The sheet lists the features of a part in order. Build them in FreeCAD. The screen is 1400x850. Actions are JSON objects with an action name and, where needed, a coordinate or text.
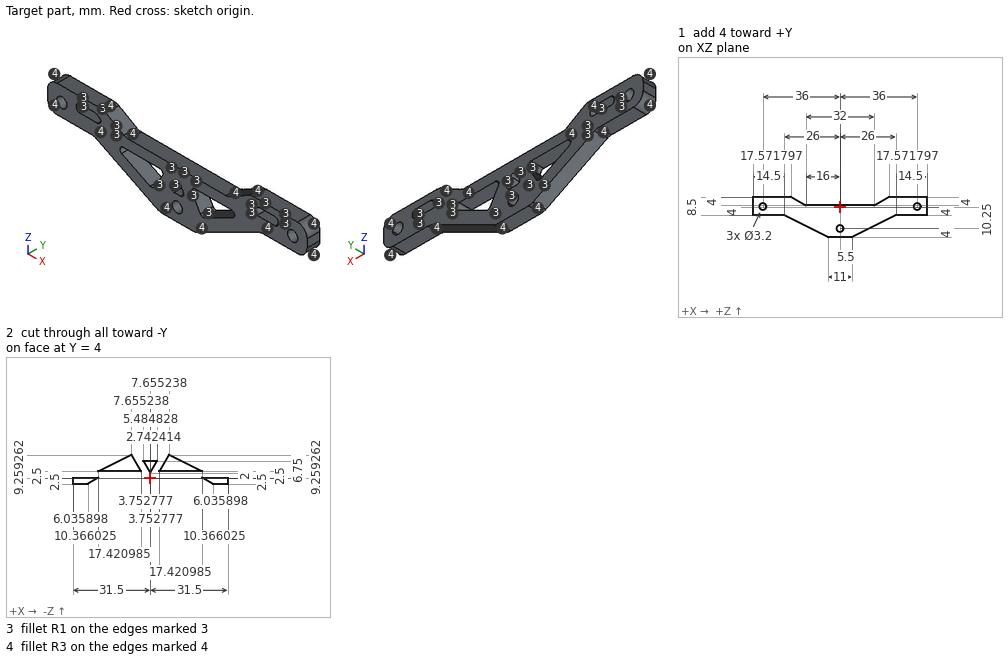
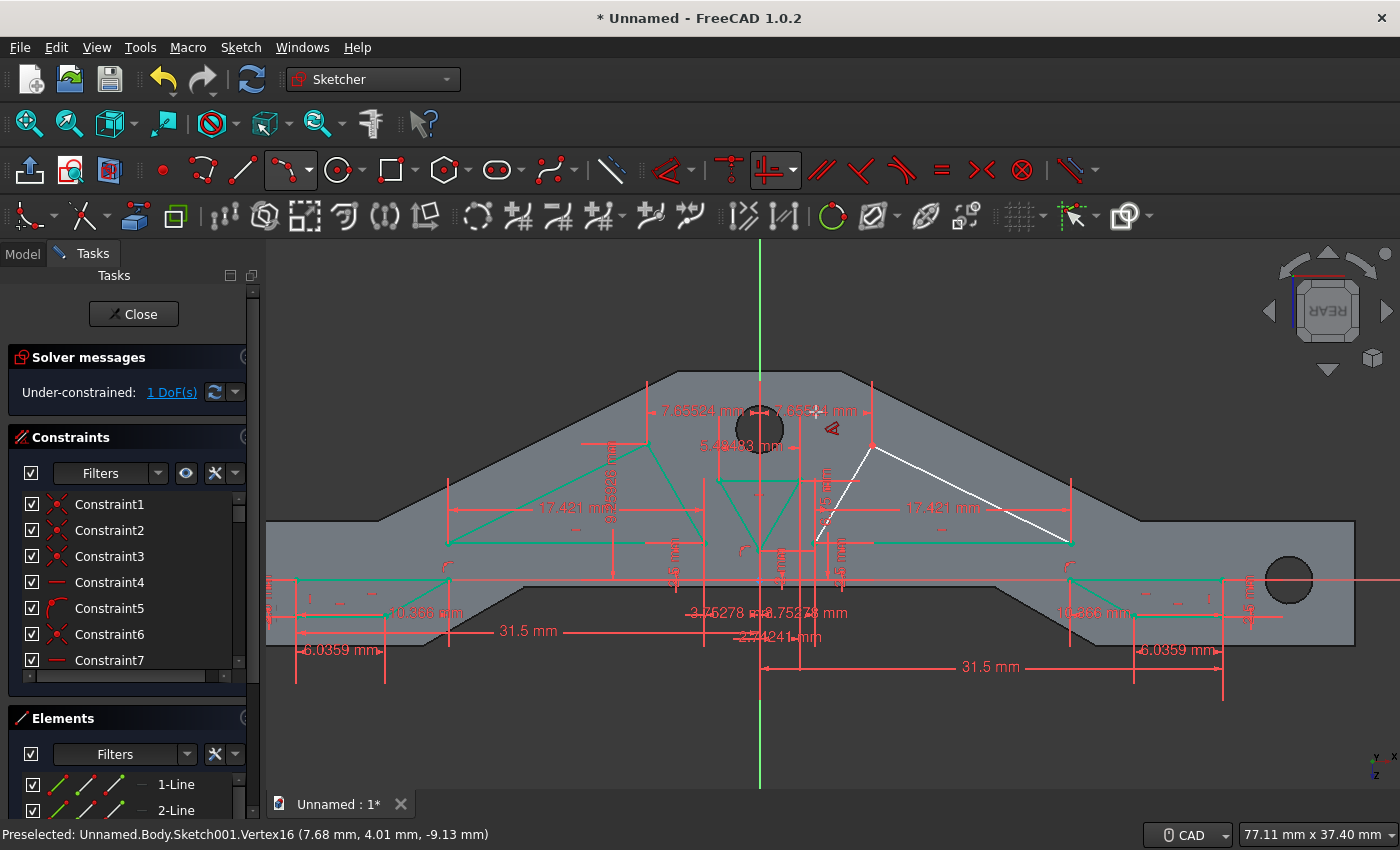
{"action": "left_click", "coordinate": [872, 446]}
{"action": "left_click", "coordinate": [906, 482]}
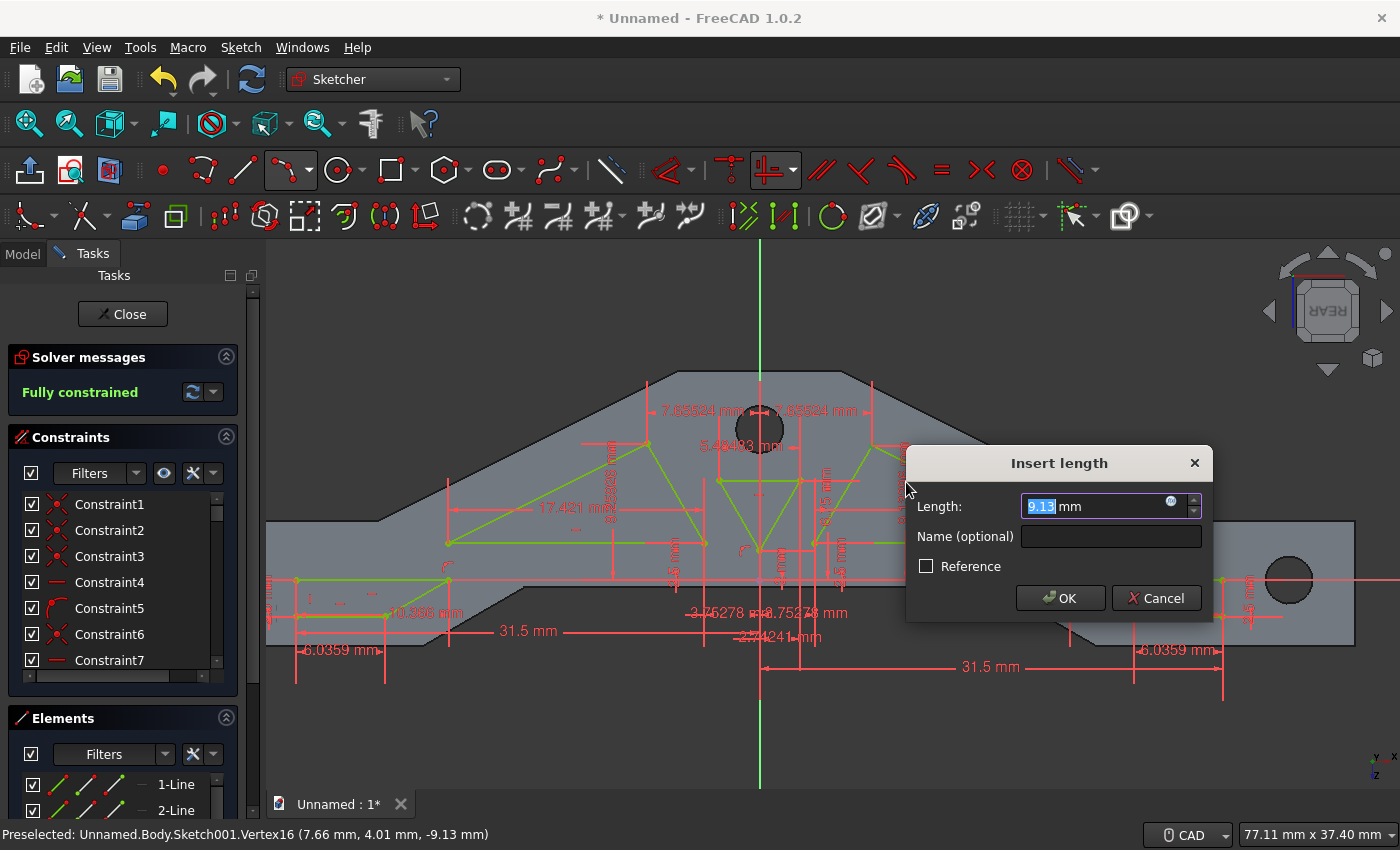
{"action": "type", "text": "9.259262"}
{"action": "key", "text": "Return"}
{"action": "key", "text": "Escape"}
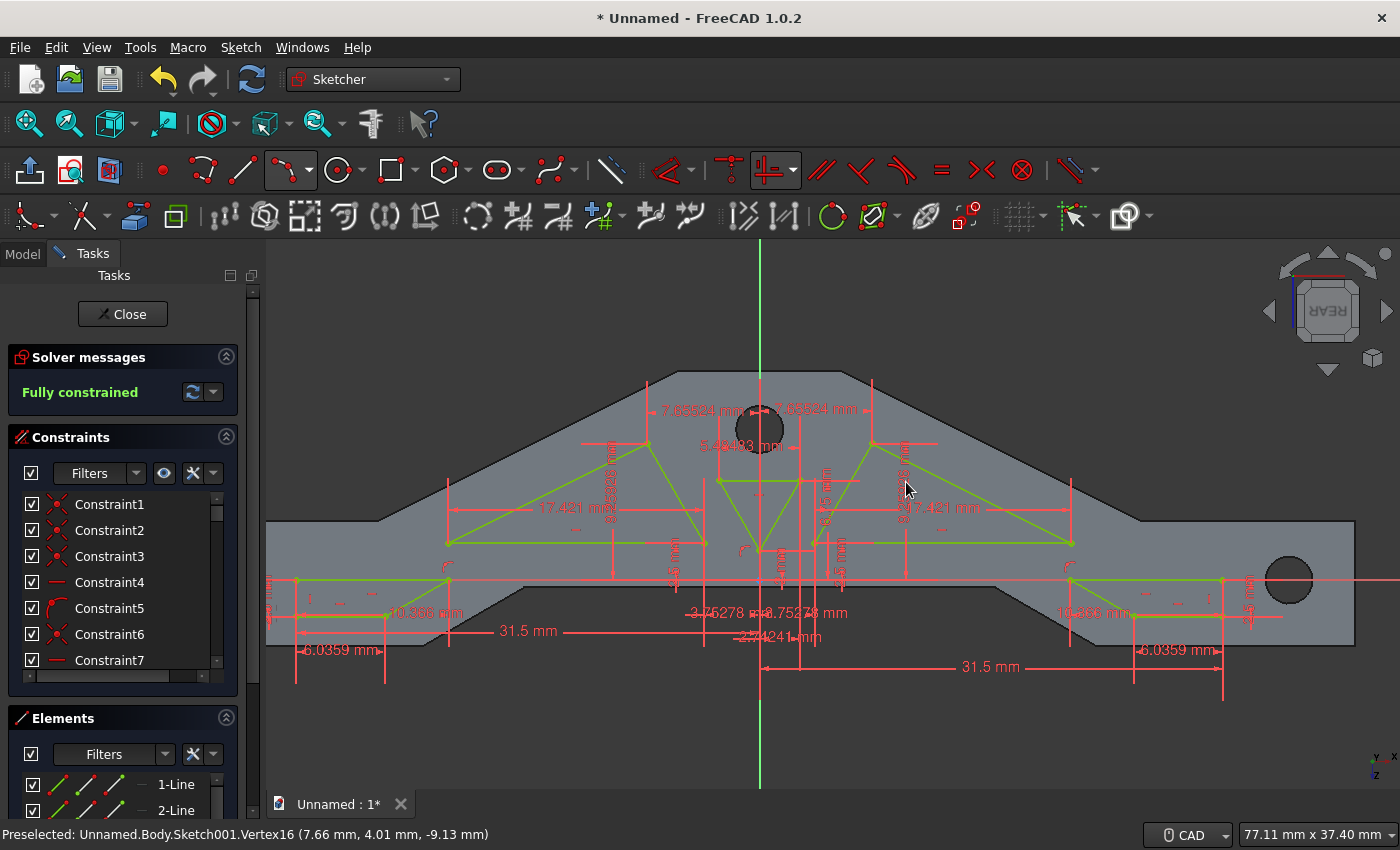
{"action": "left_click", "coordinate": [123, 314]}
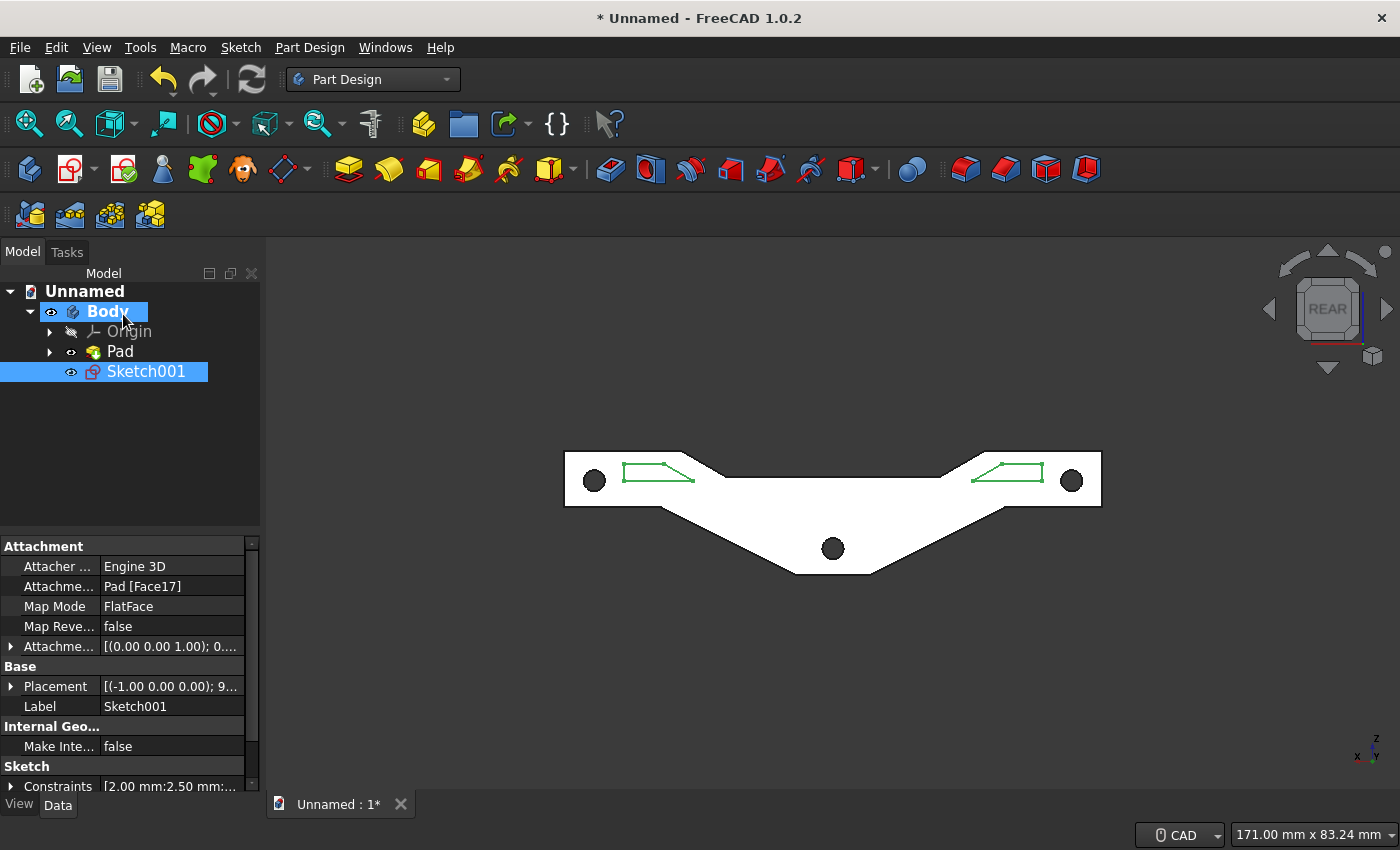
{"action": "left_click", "coordinate": [612, 170]}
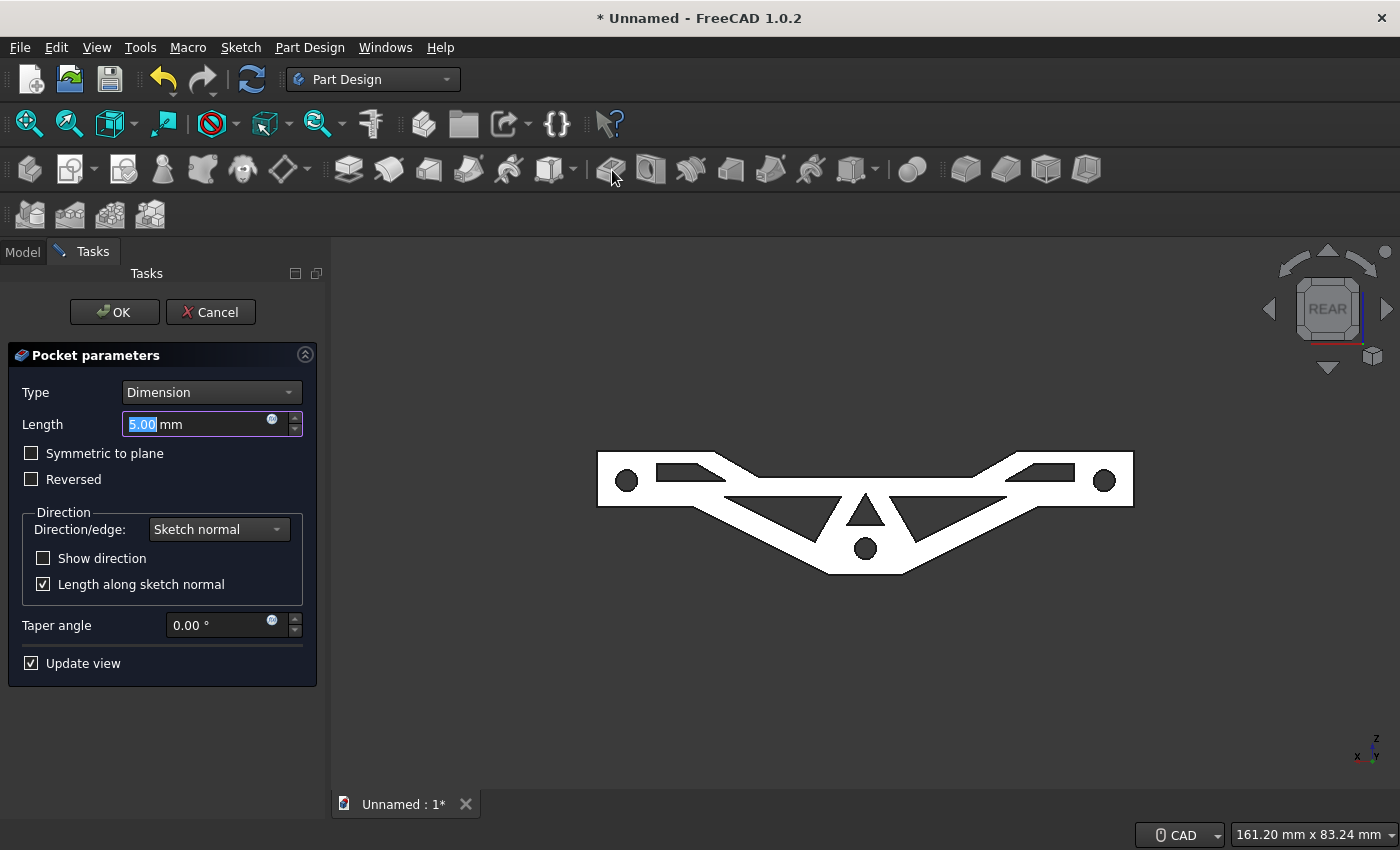
{"action": "left_click", "coordinate": [212, 392]}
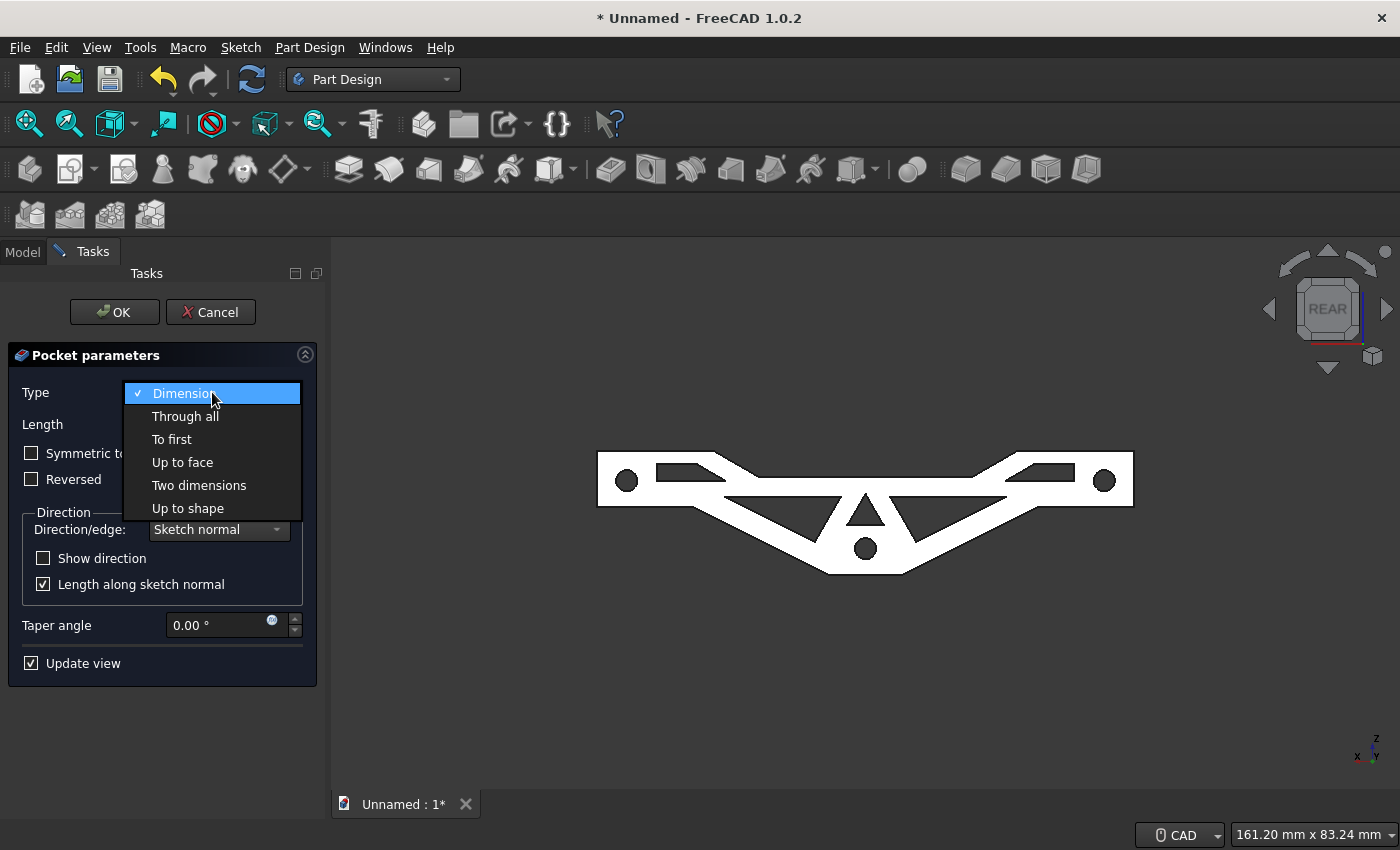
{"action": "left_click", "coordinate": [212, 416]}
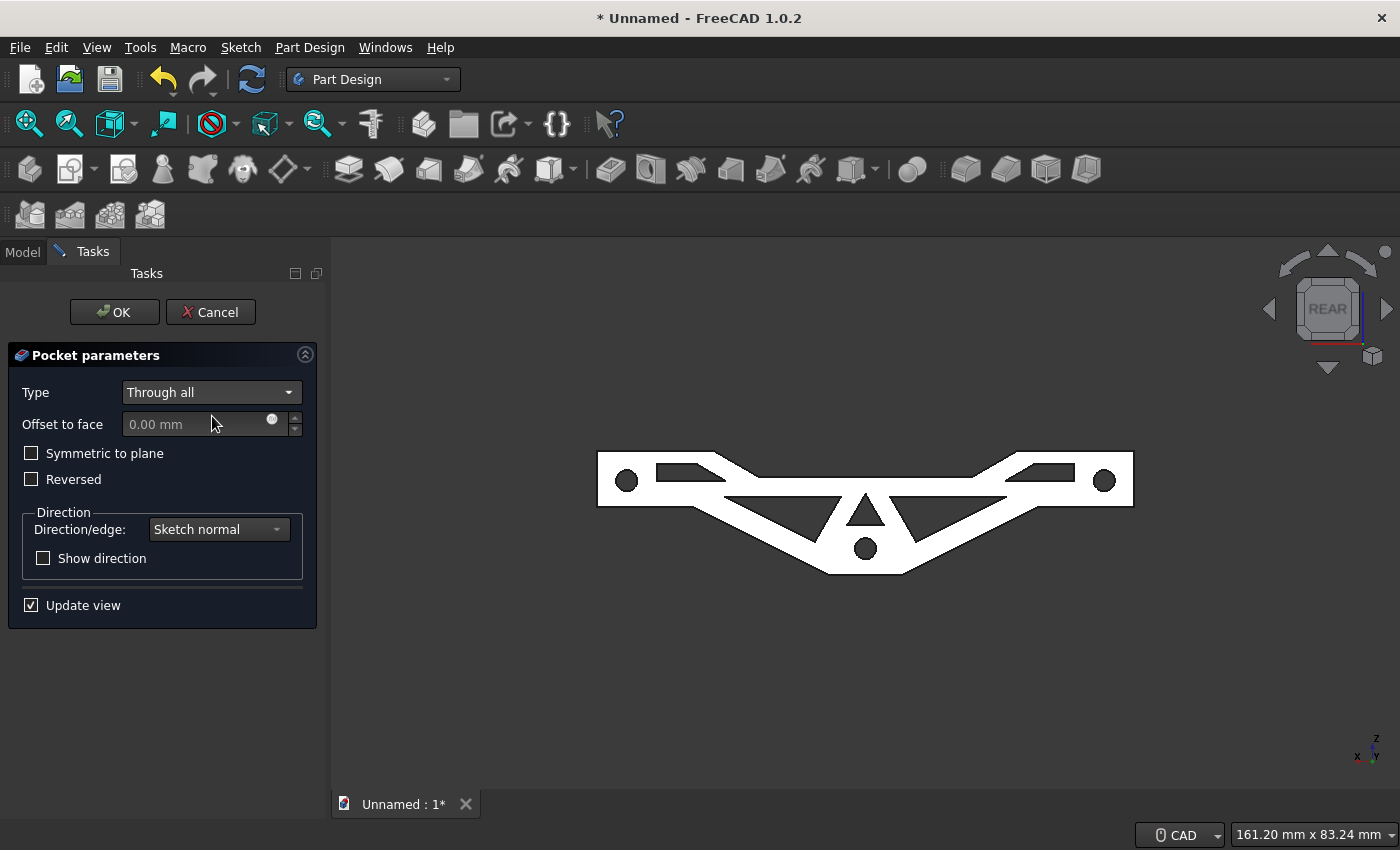
{"action": "left_click", "coordinate": [115, 312]}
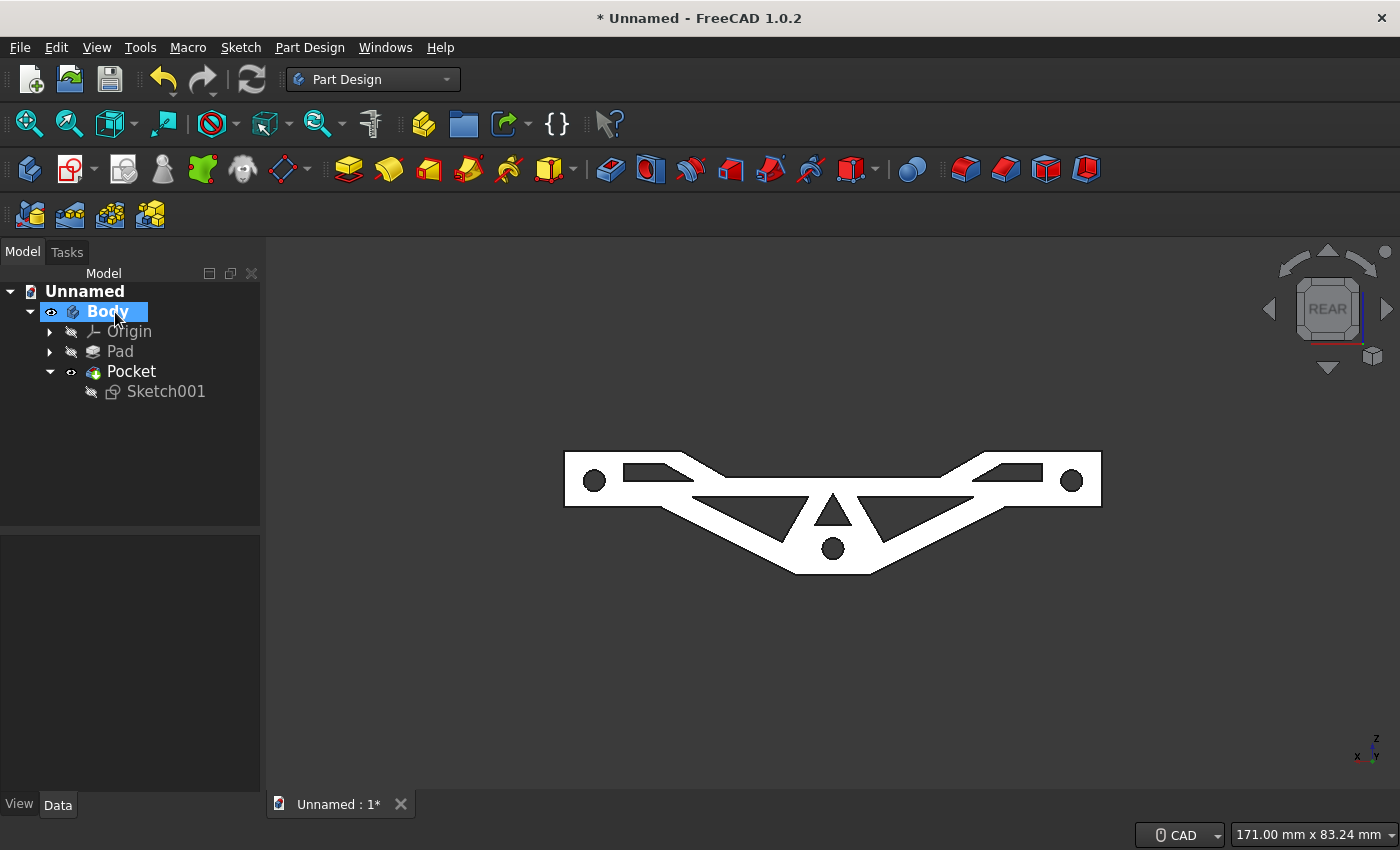
{"action": "key", "text": "0"}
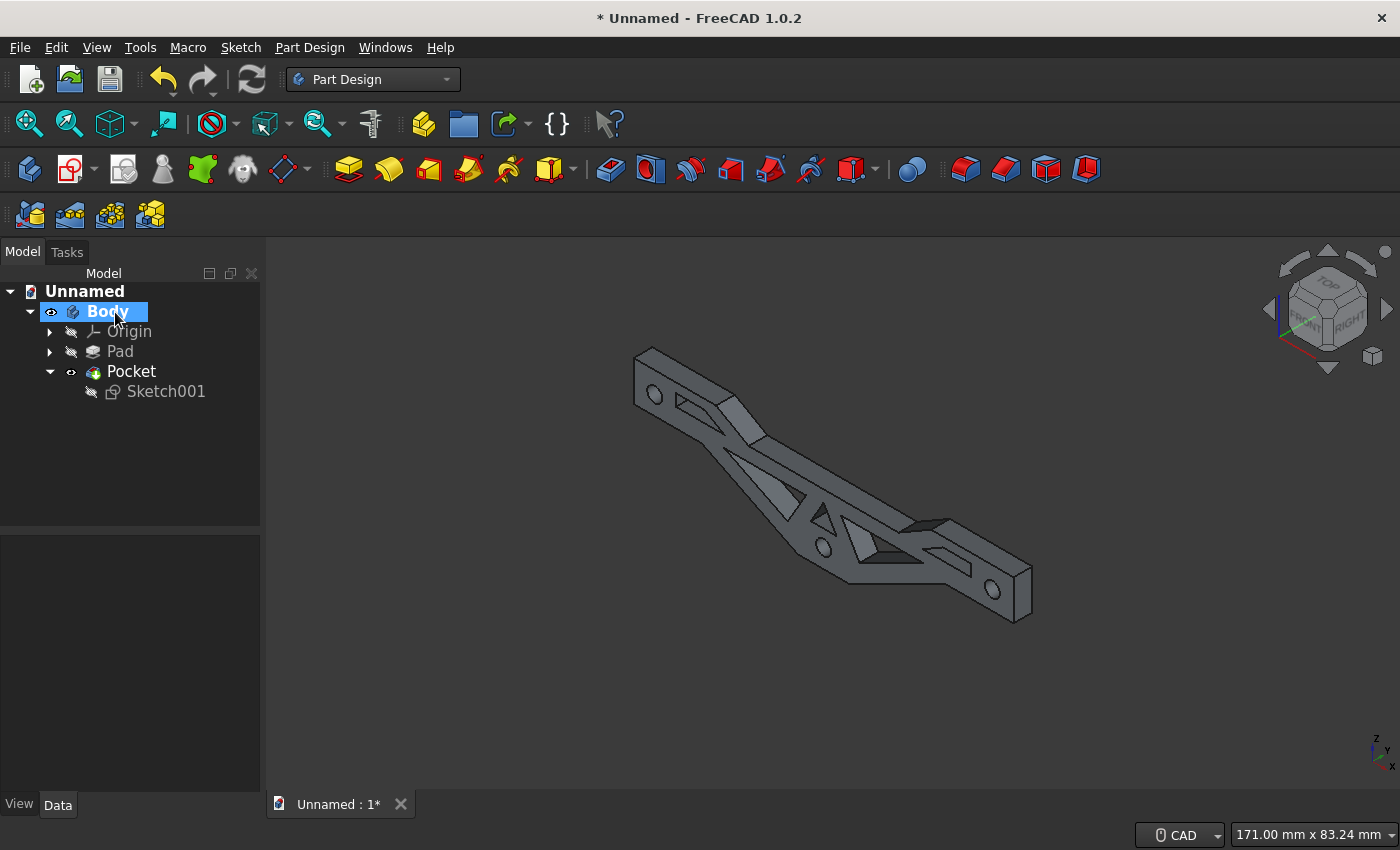
{"action": "key", "text": "2"}